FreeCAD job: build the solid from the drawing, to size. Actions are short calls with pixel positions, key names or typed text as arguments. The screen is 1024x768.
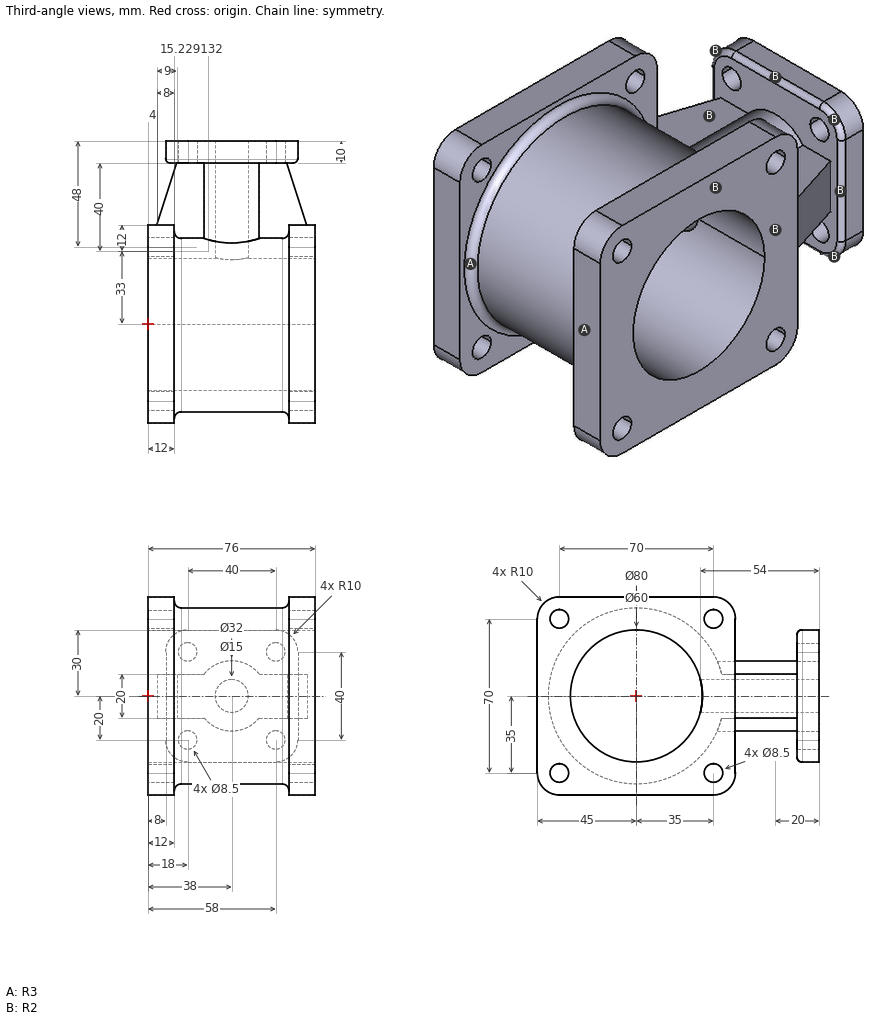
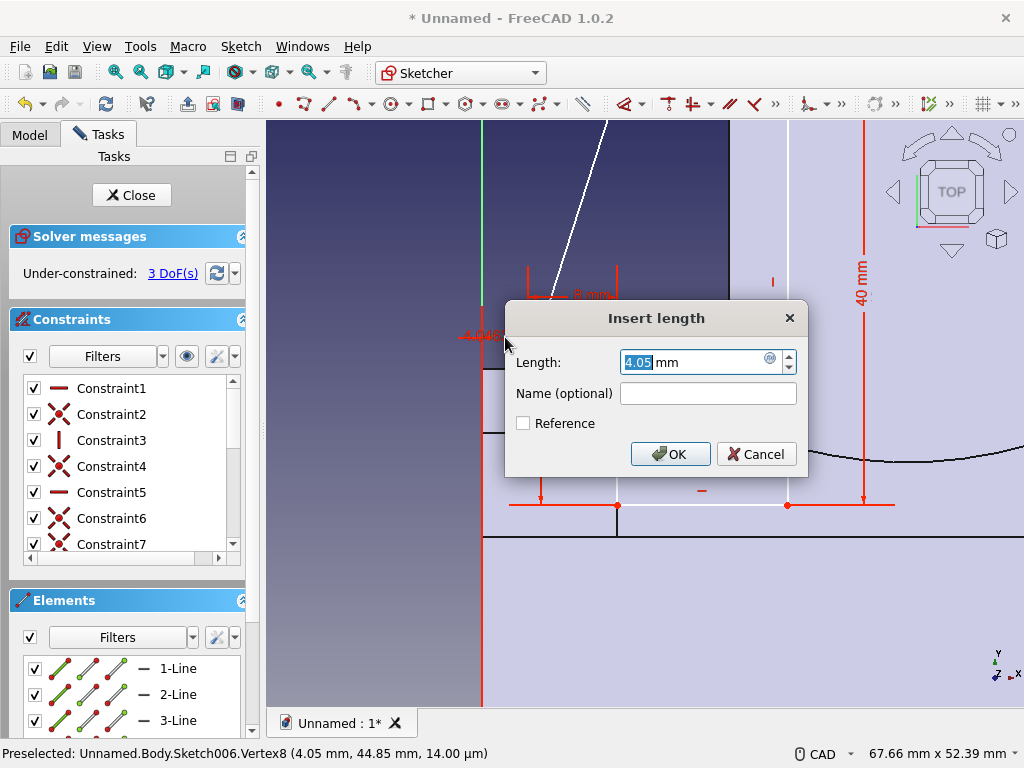
text(4)
key(Return)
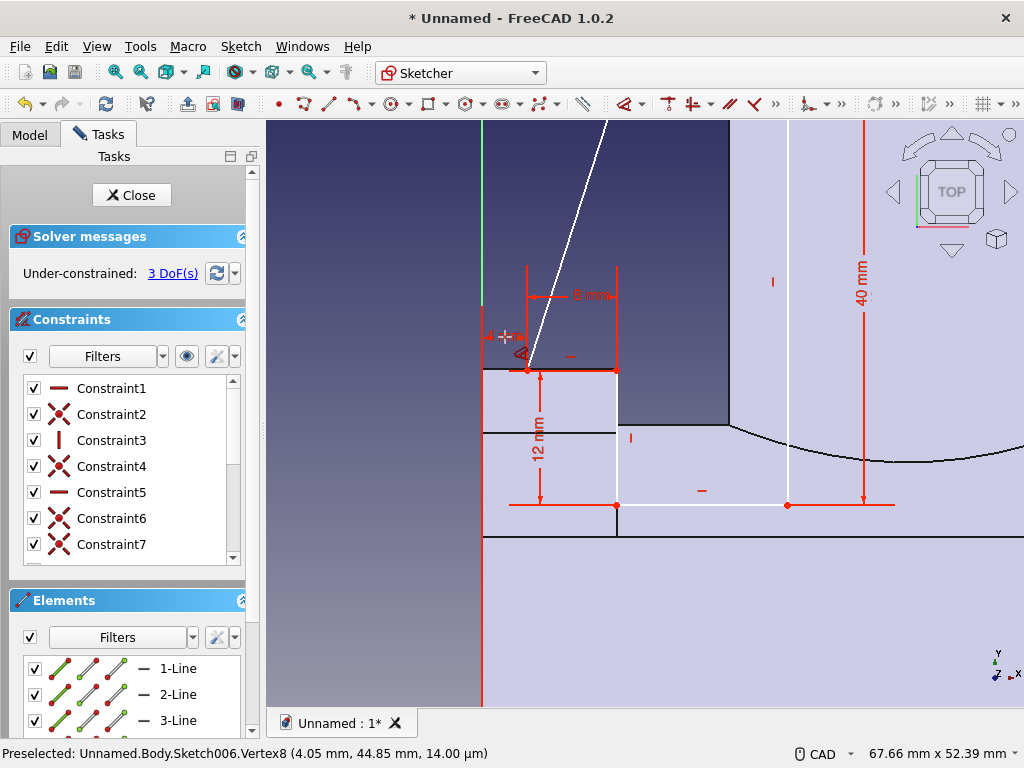
click(598, 151)
click(577, 405)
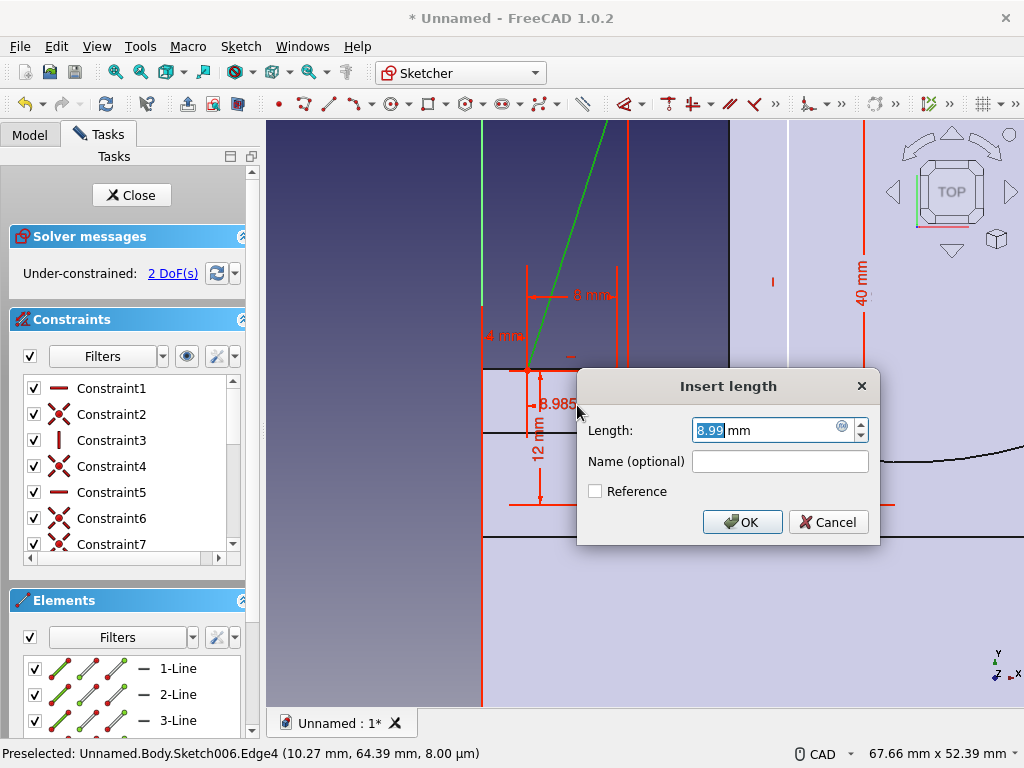
text(9)
key(Return)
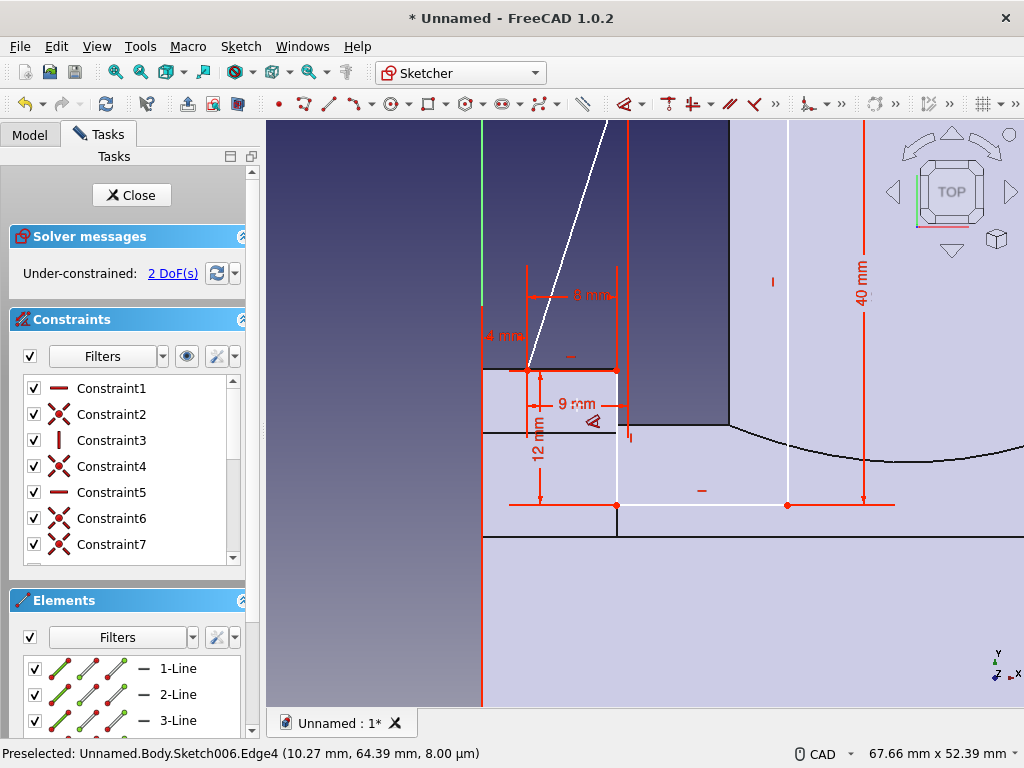
click(617, 505)
click(448, 592)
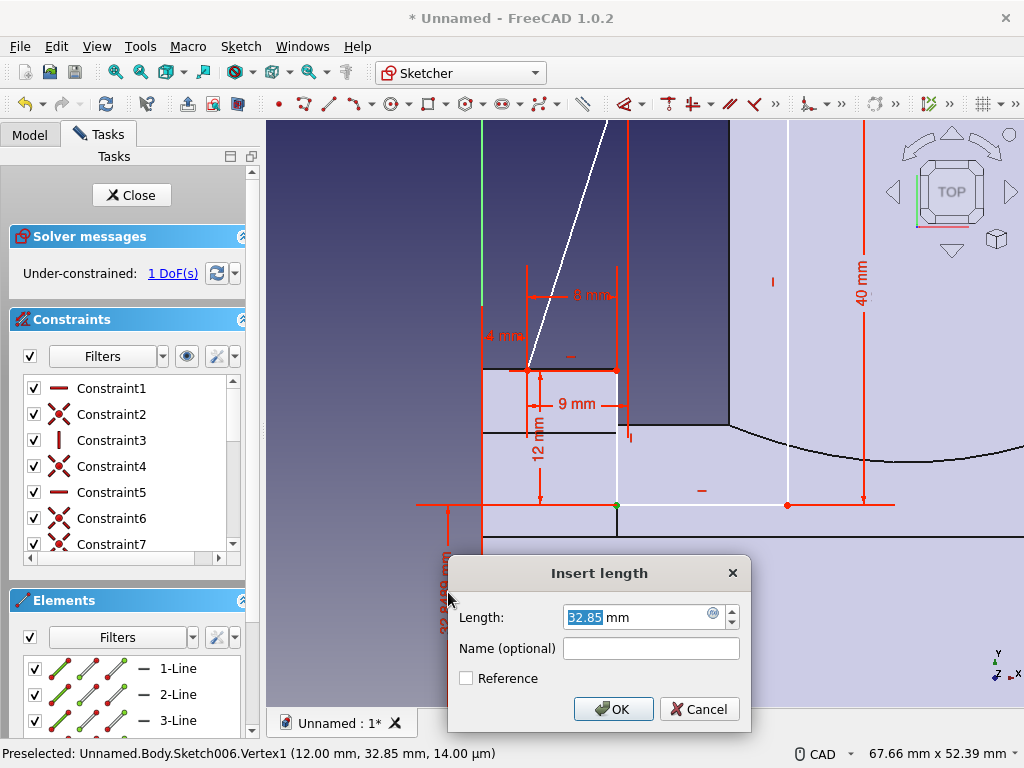
text(33)
key(Return)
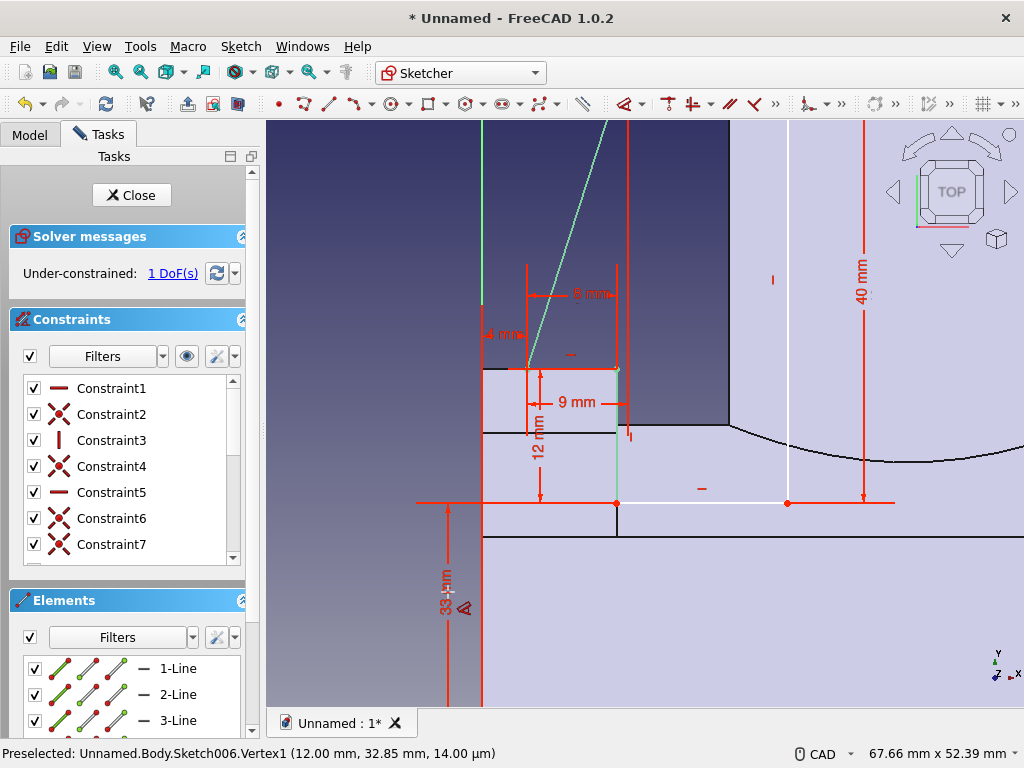
click(668, 503)
click(702, 537)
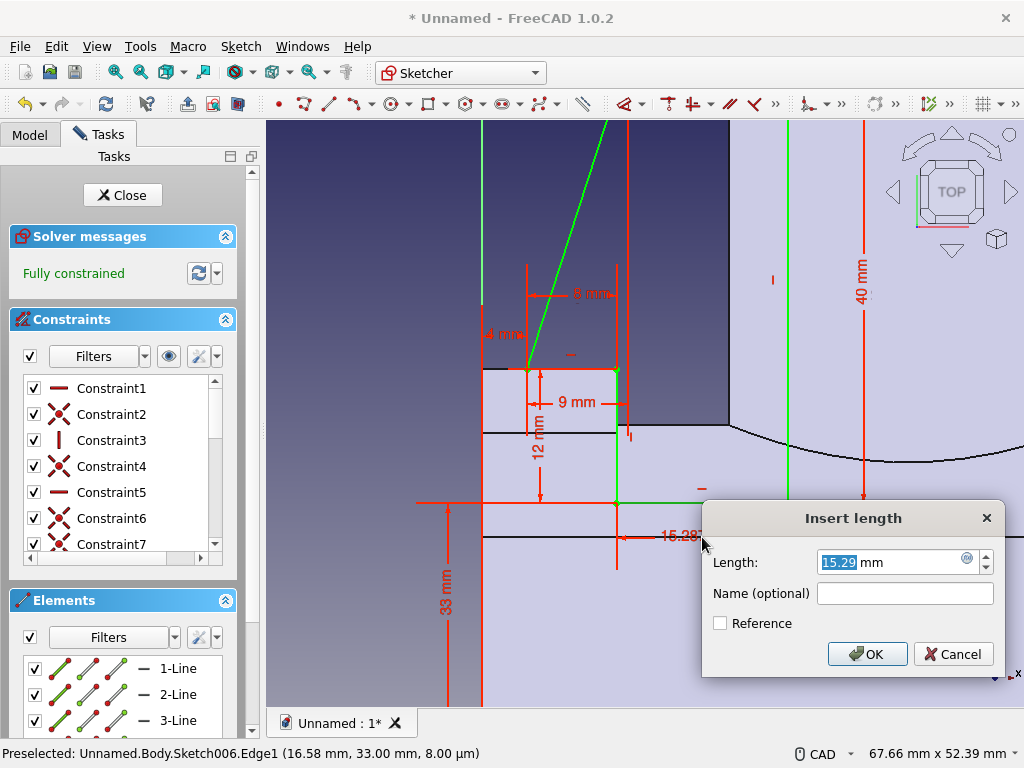
text(15.229132)
key(Return)
key(Escape)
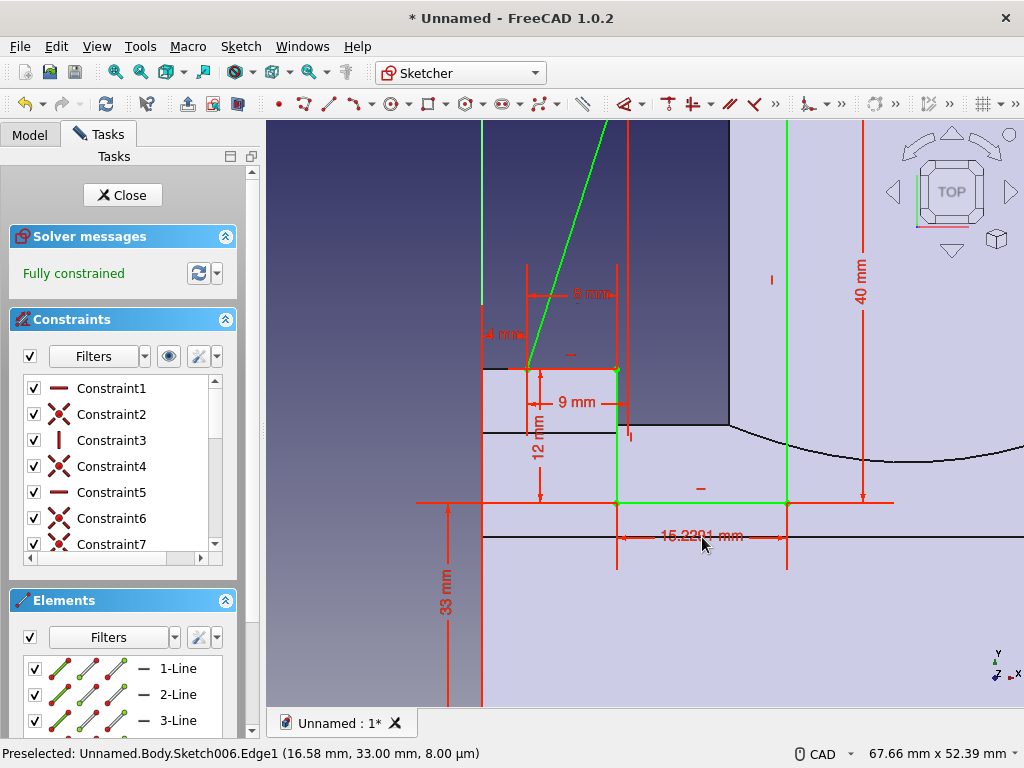
click(123, 195)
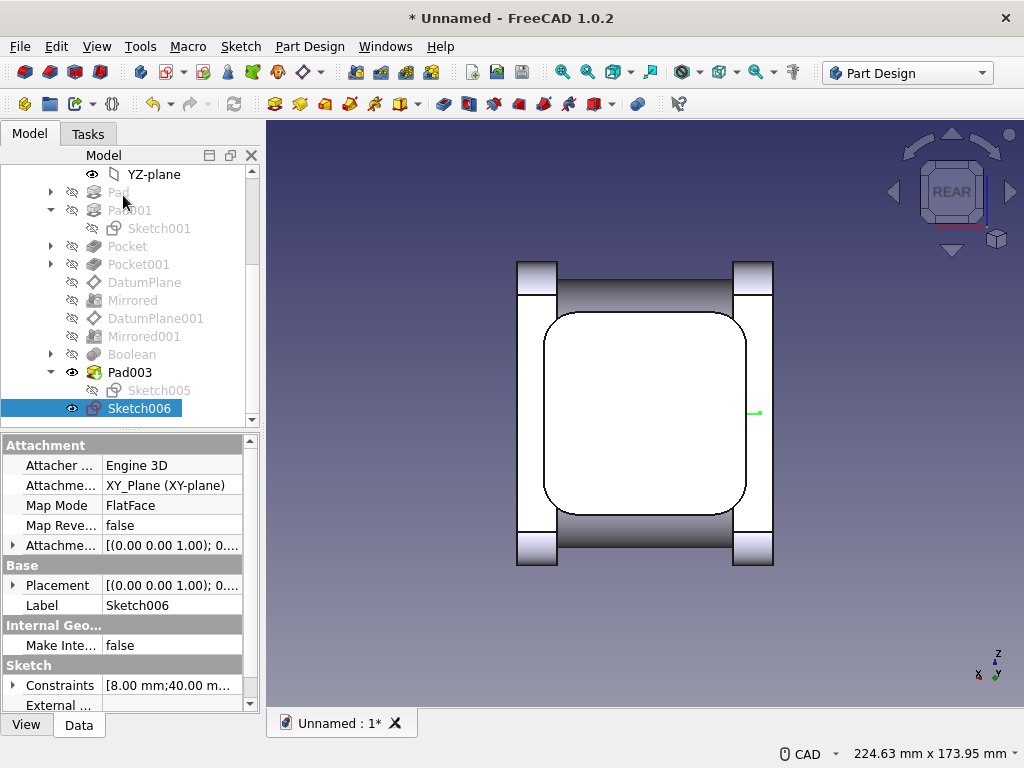
click(275, 104)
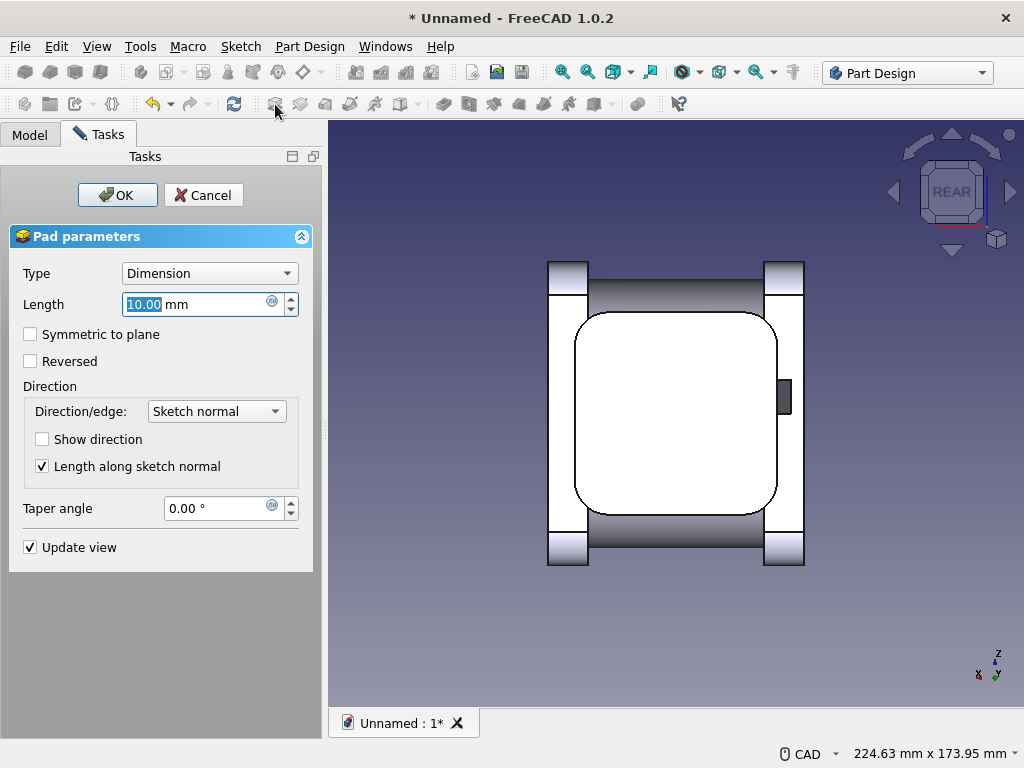
text(20)
key(Tab)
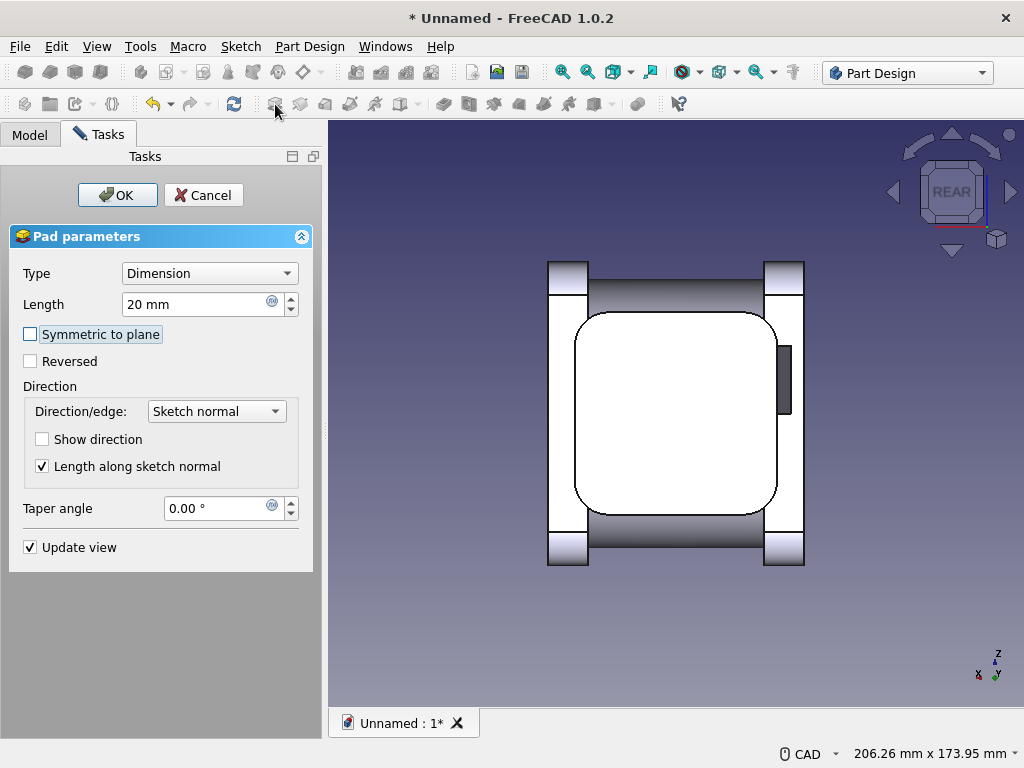
click(31, 334)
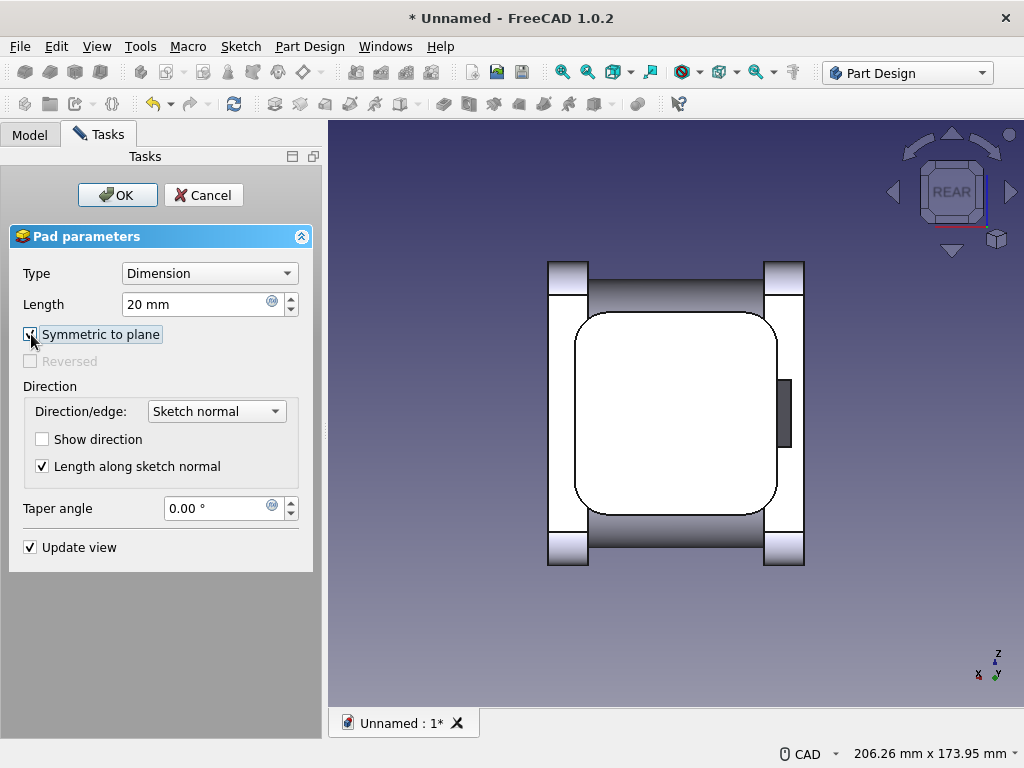
click(118, 195)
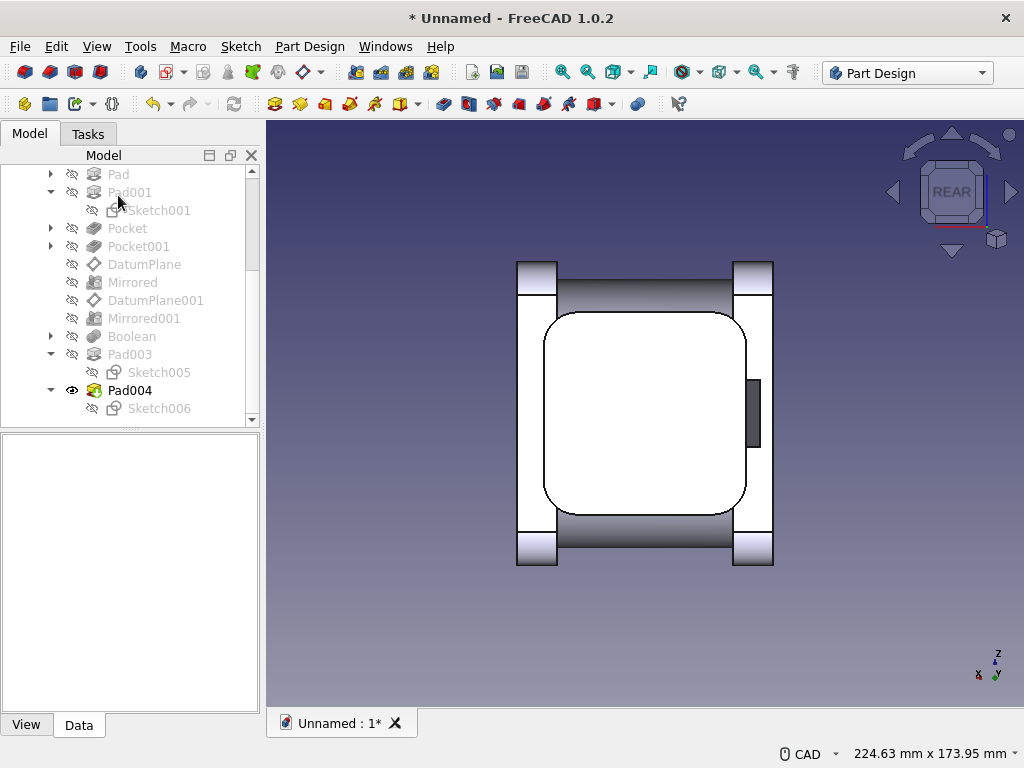
scroll(141, 296, down, 3)